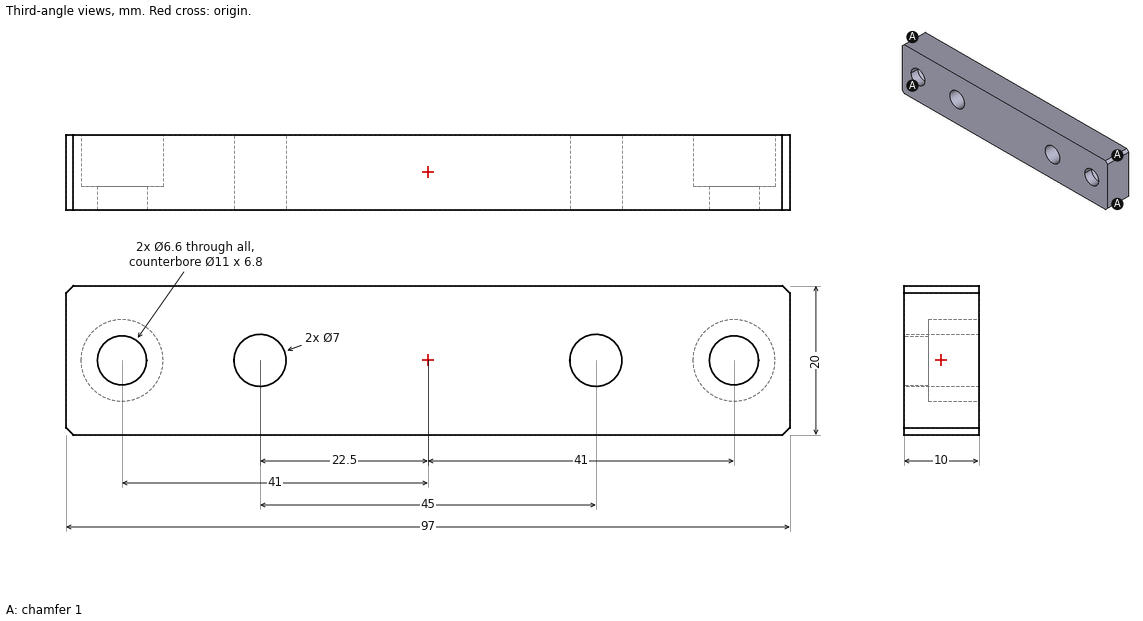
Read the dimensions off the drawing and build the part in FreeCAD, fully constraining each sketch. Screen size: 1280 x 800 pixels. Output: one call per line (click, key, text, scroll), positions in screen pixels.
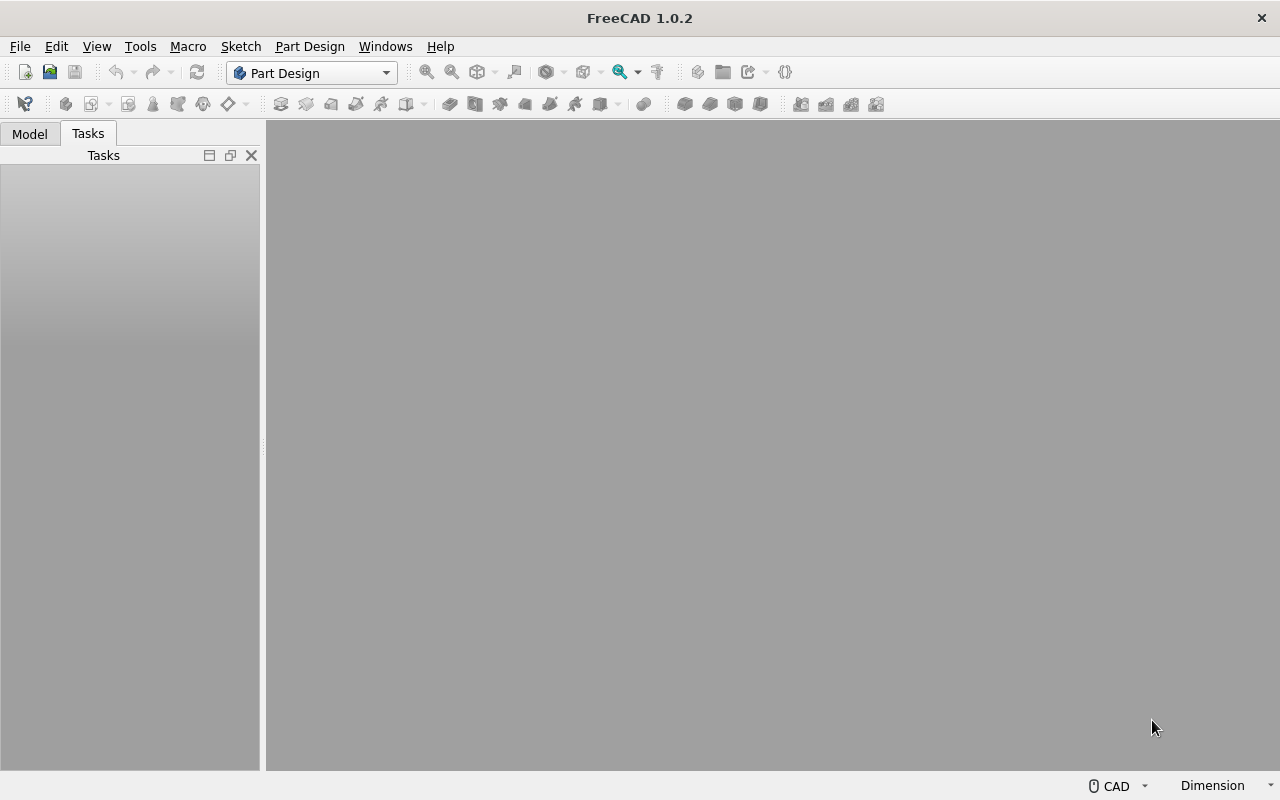
click(25, 72)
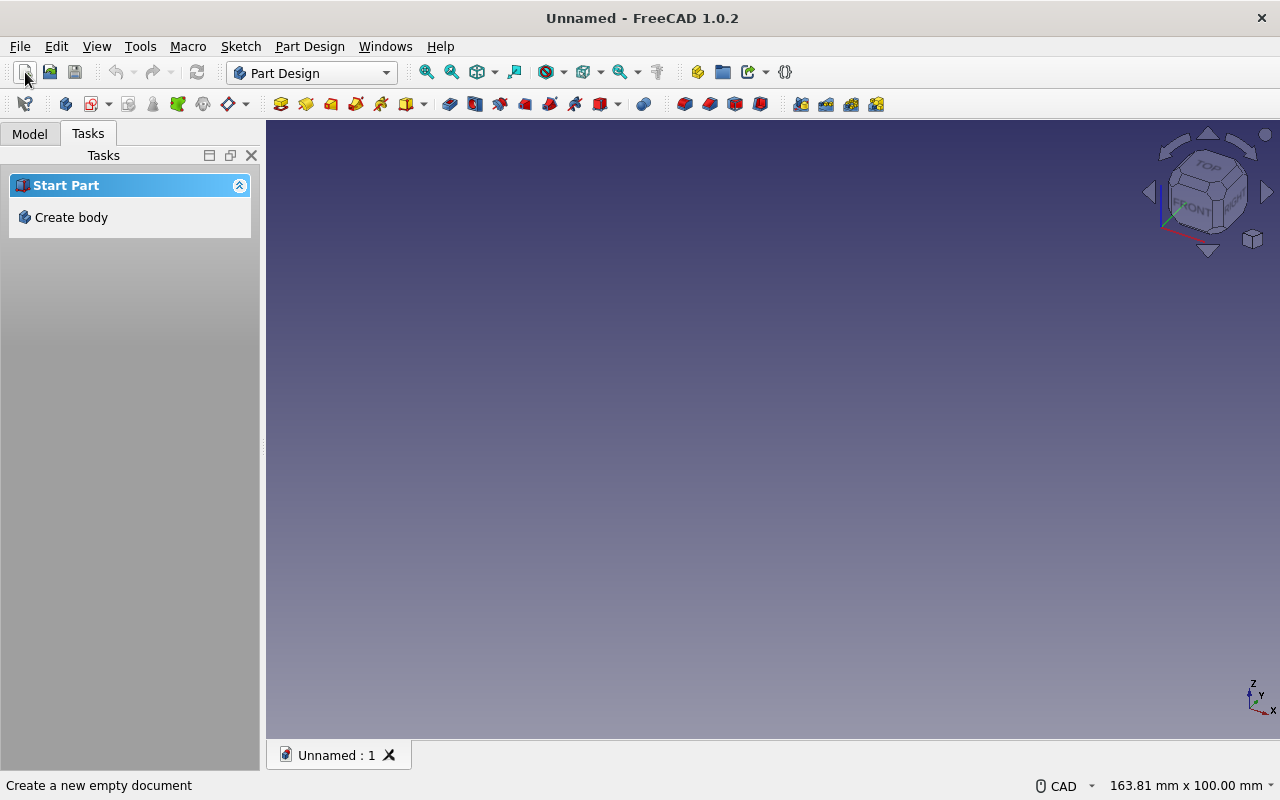
click(90, 104)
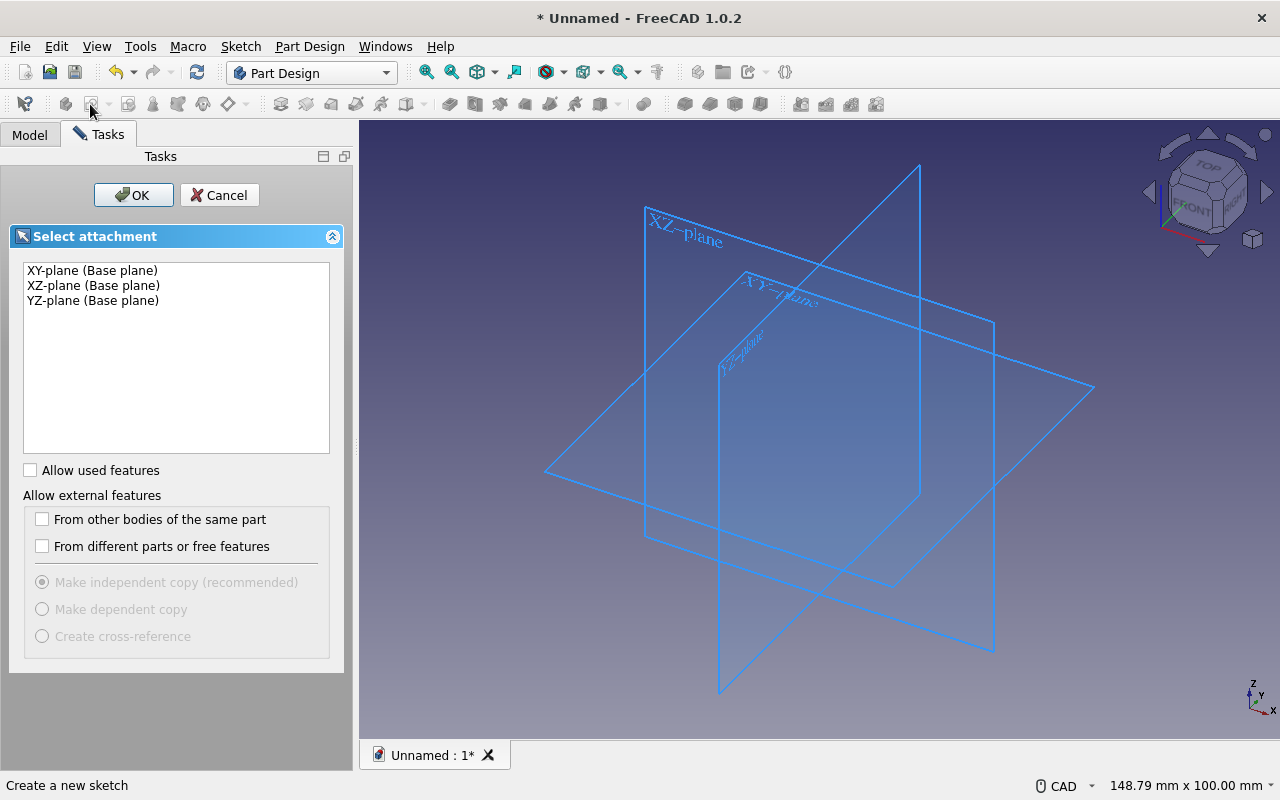
click(84, 286)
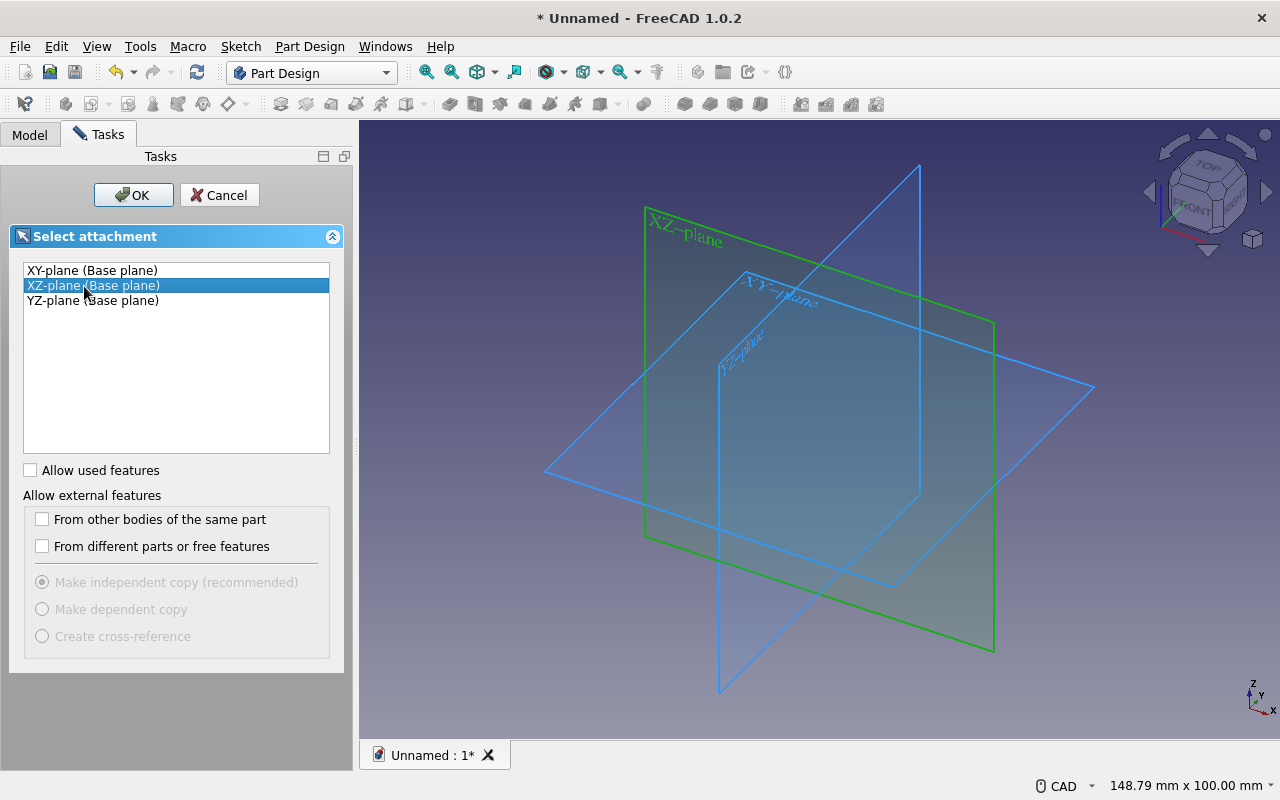
click(134, 195)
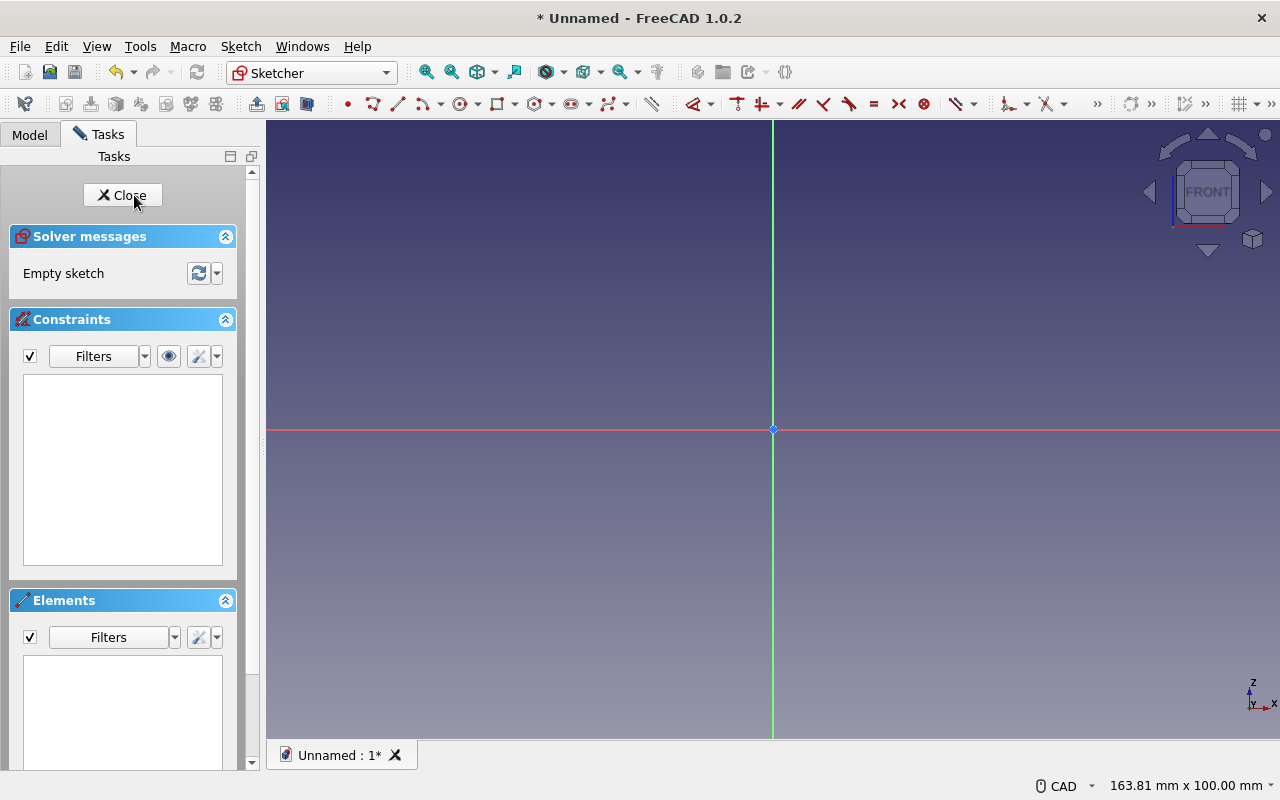
key(g)
key(v)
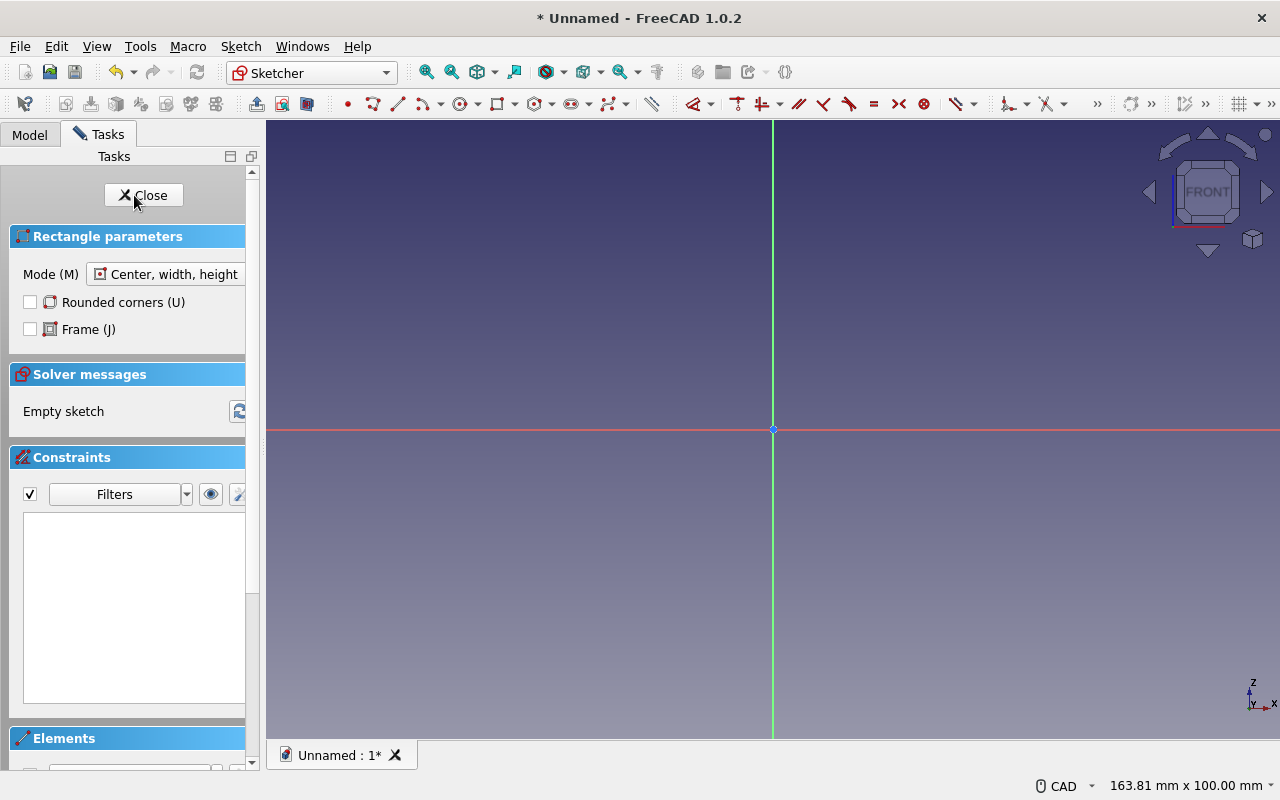
click(773, 430)
click(1073, 368)
key(Escape)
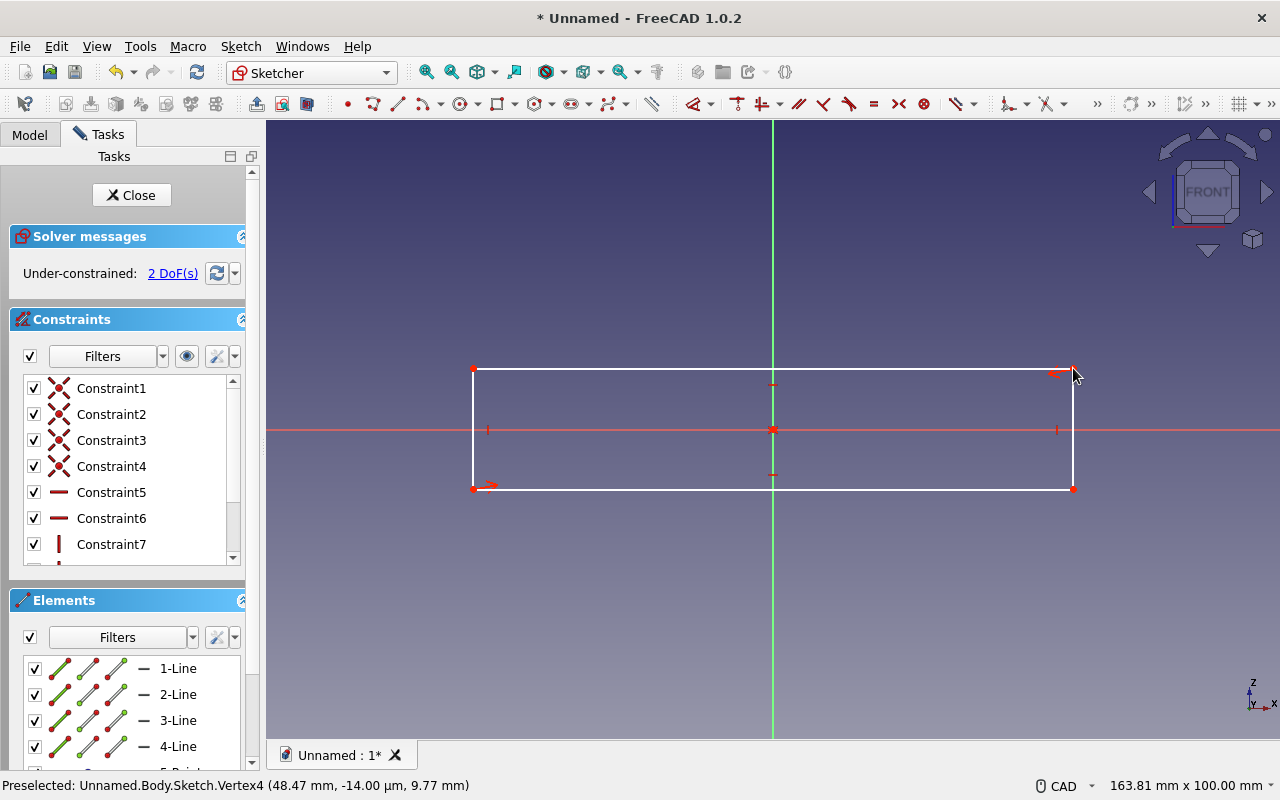
click(653, 490)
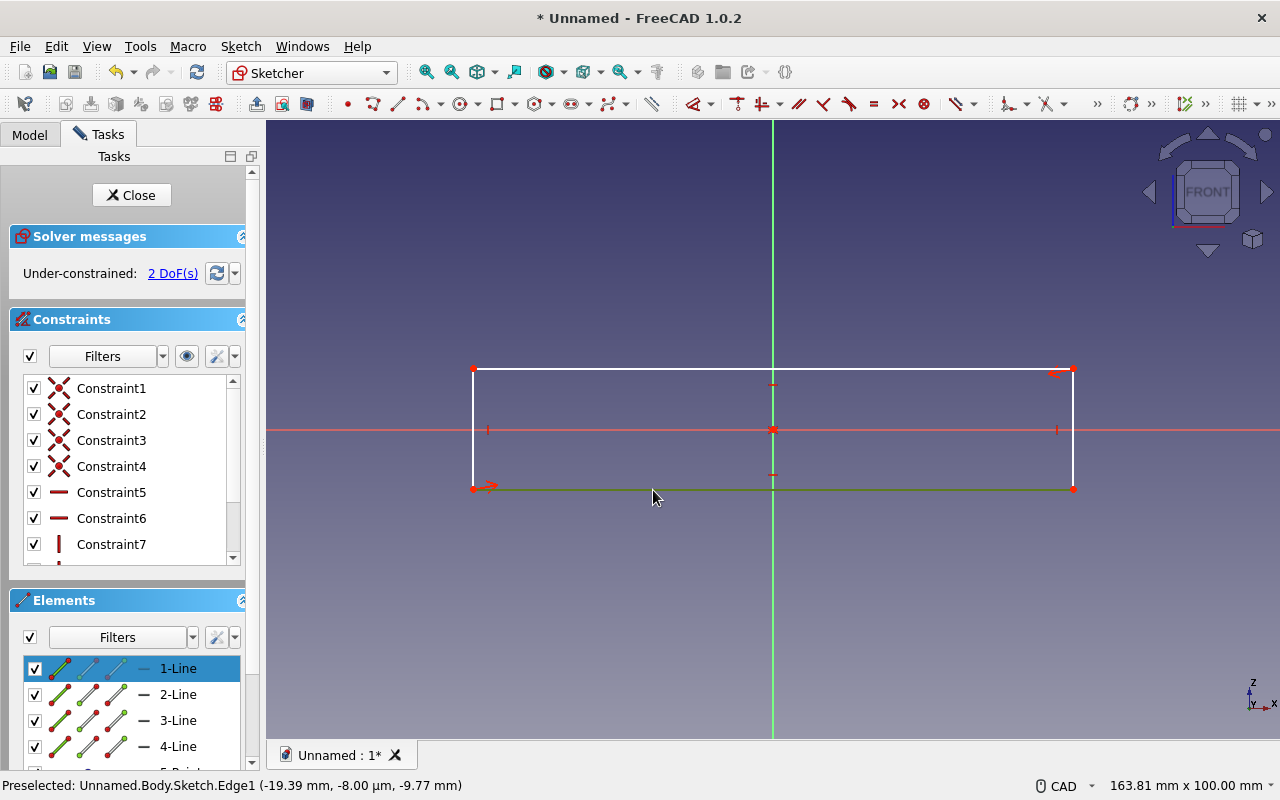
click(710, 104)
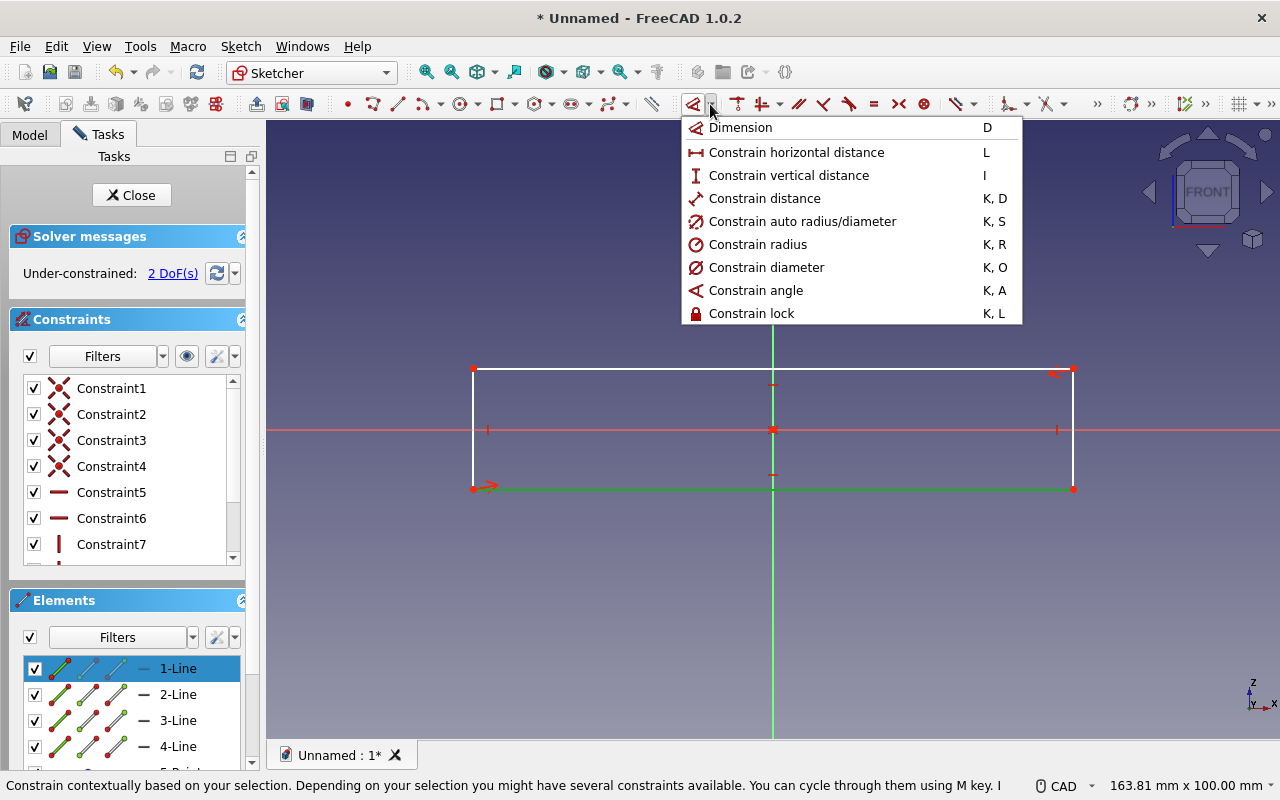
click(852, 152)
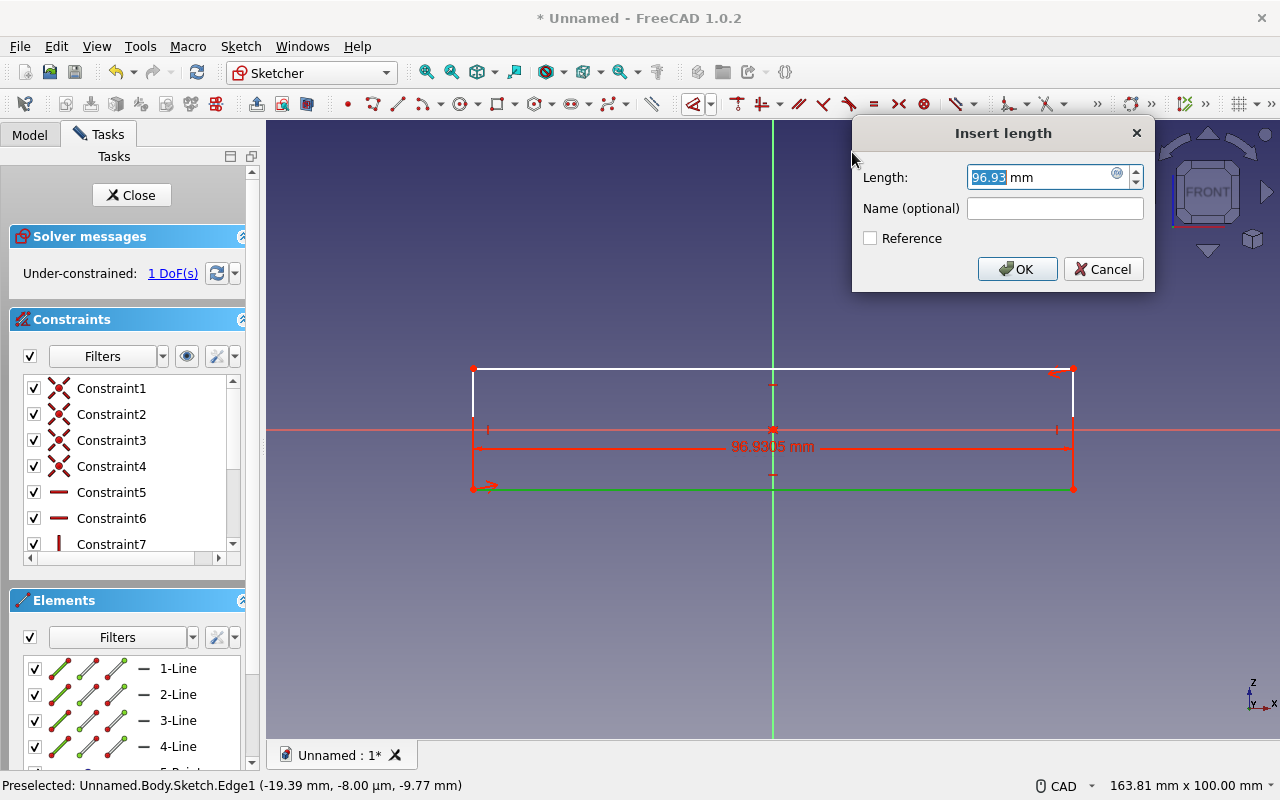
text(97)
key(Return)